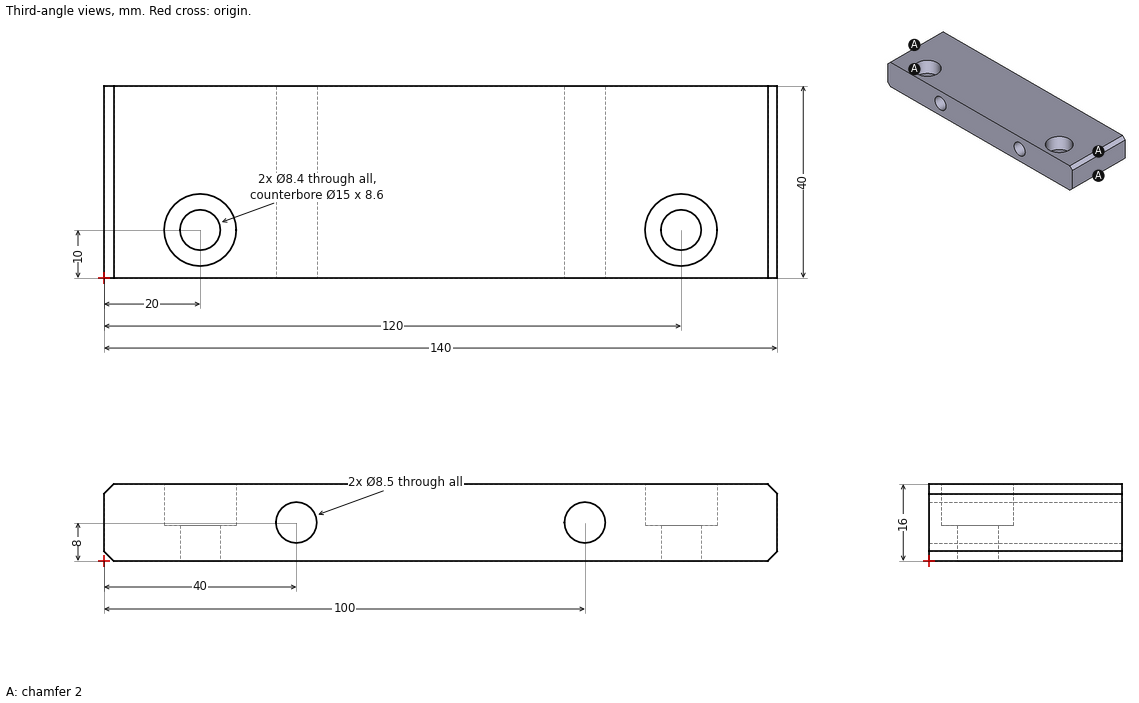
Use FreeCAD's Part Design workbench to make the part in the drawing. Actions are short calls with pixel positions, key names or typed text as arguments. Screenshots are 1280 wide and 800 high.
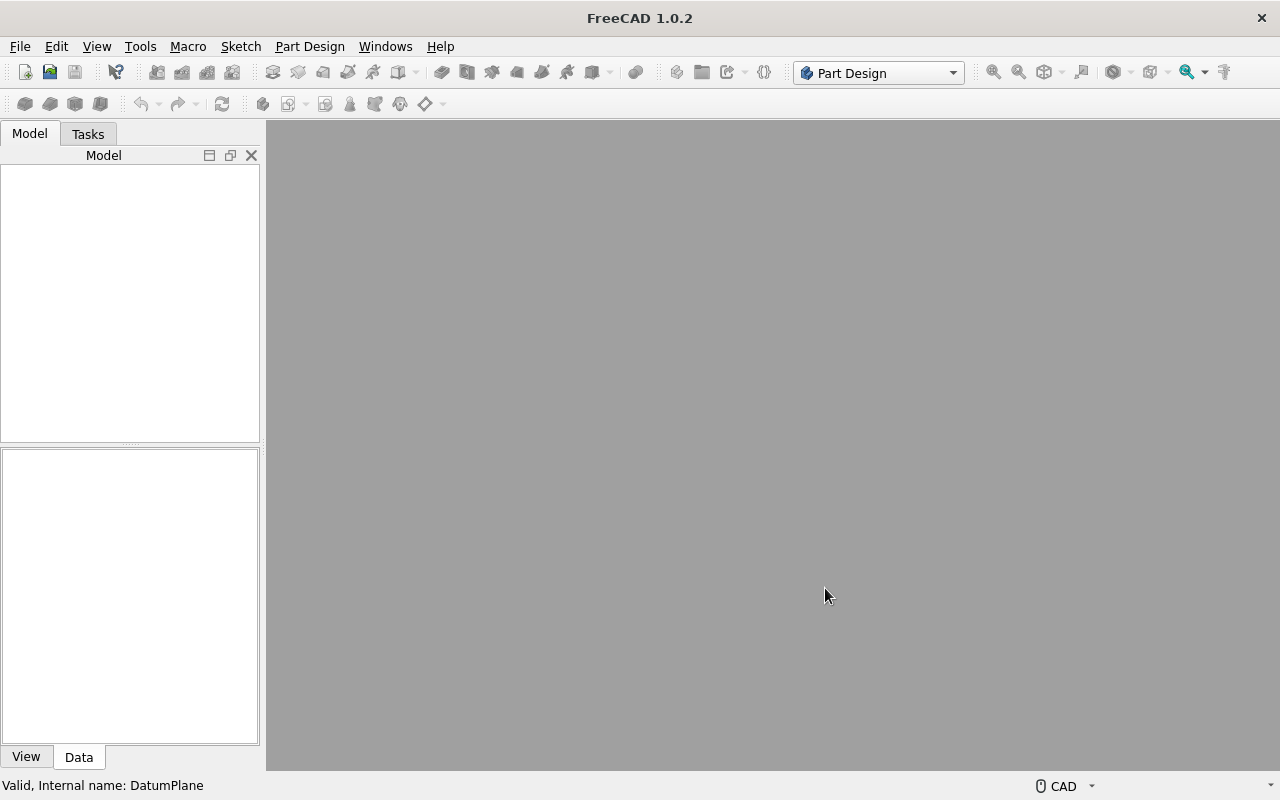
click(25, 72)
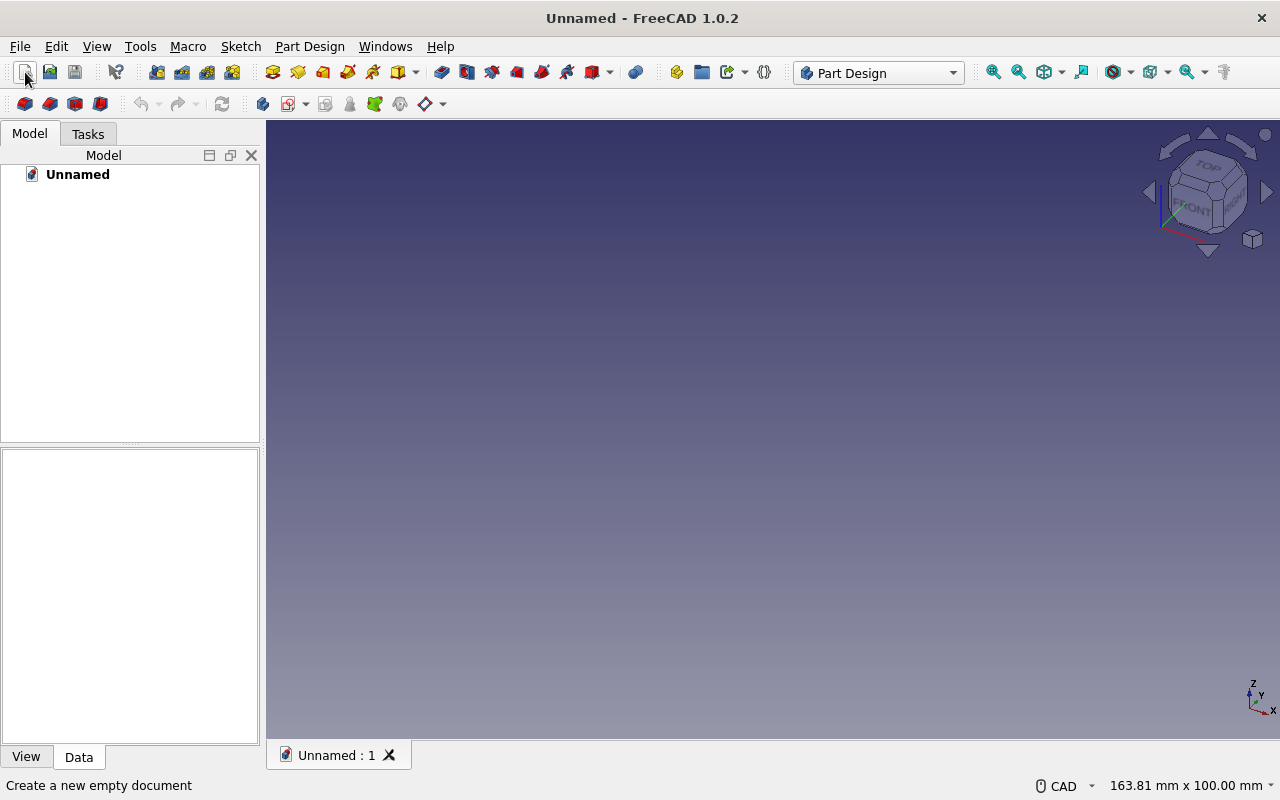
click(288, 104)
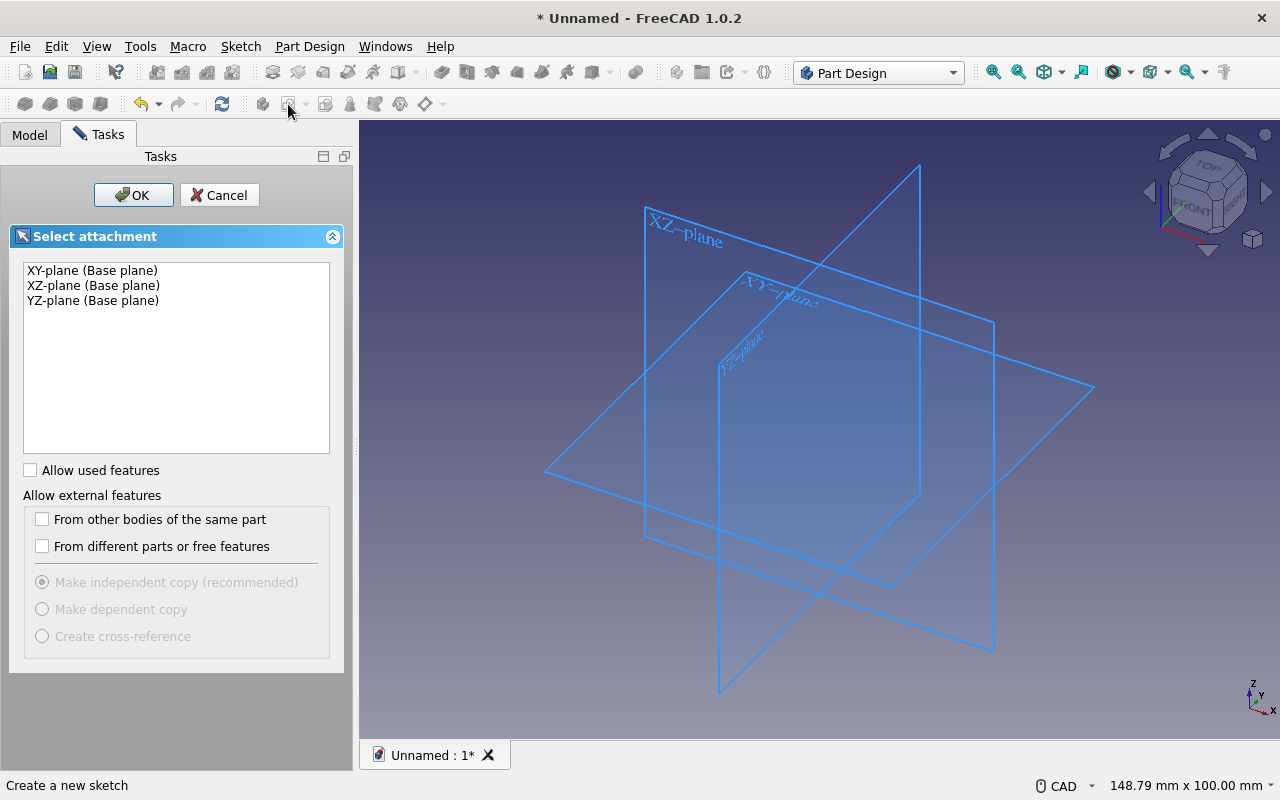
click(84, 270)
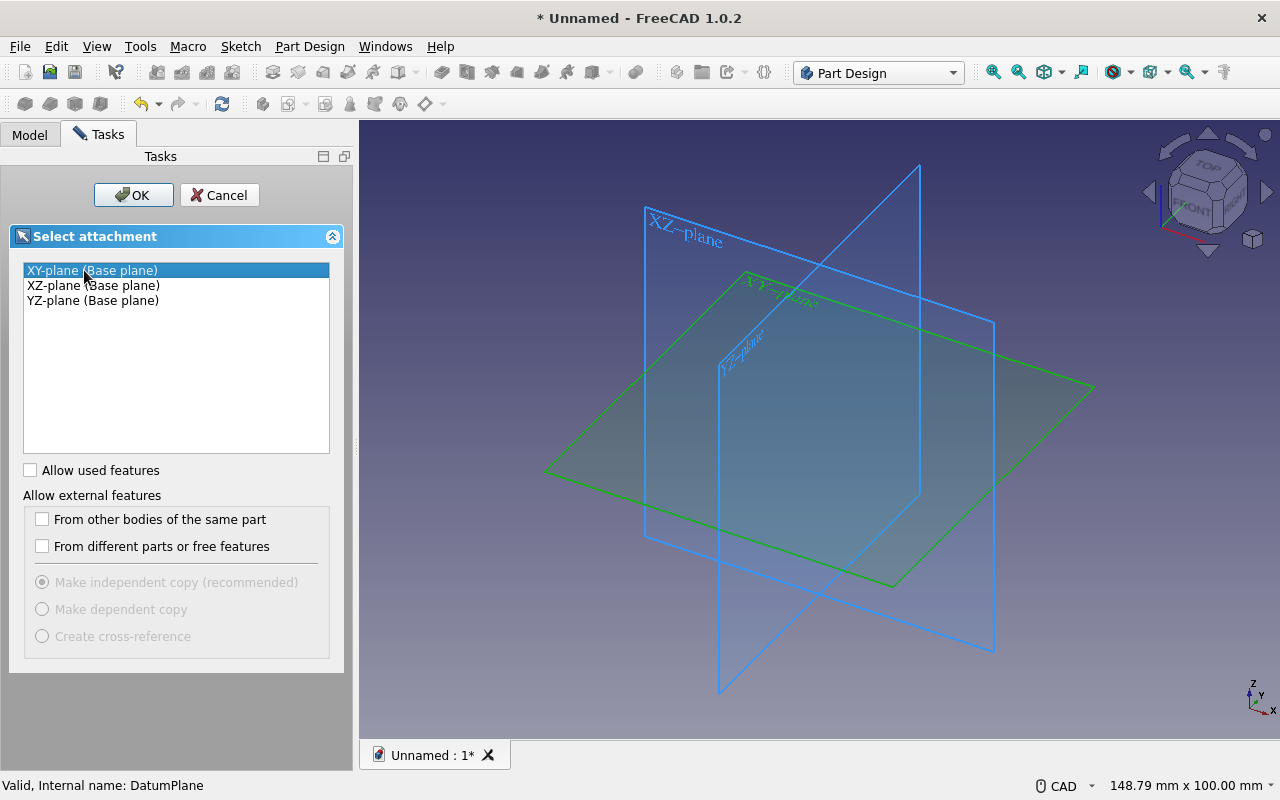
click(134, 195)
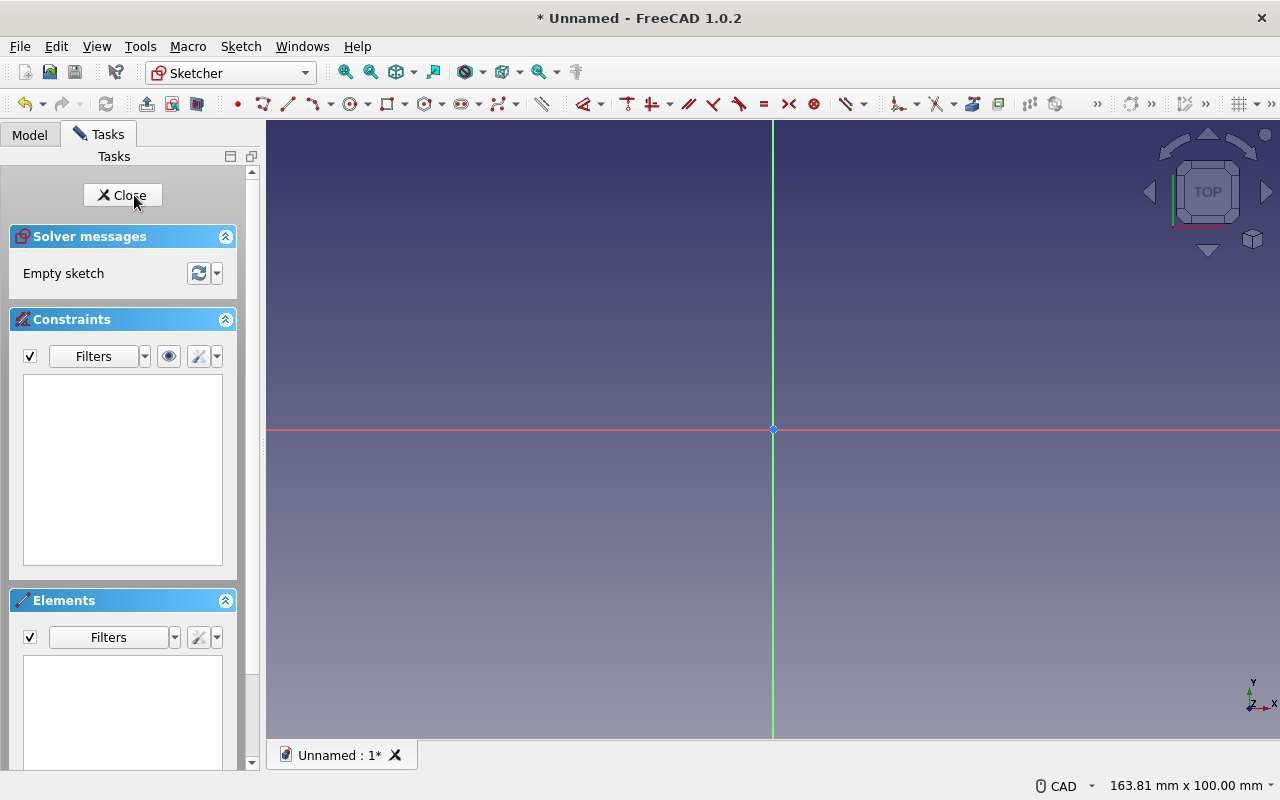
scroll(294, 580, down, 3)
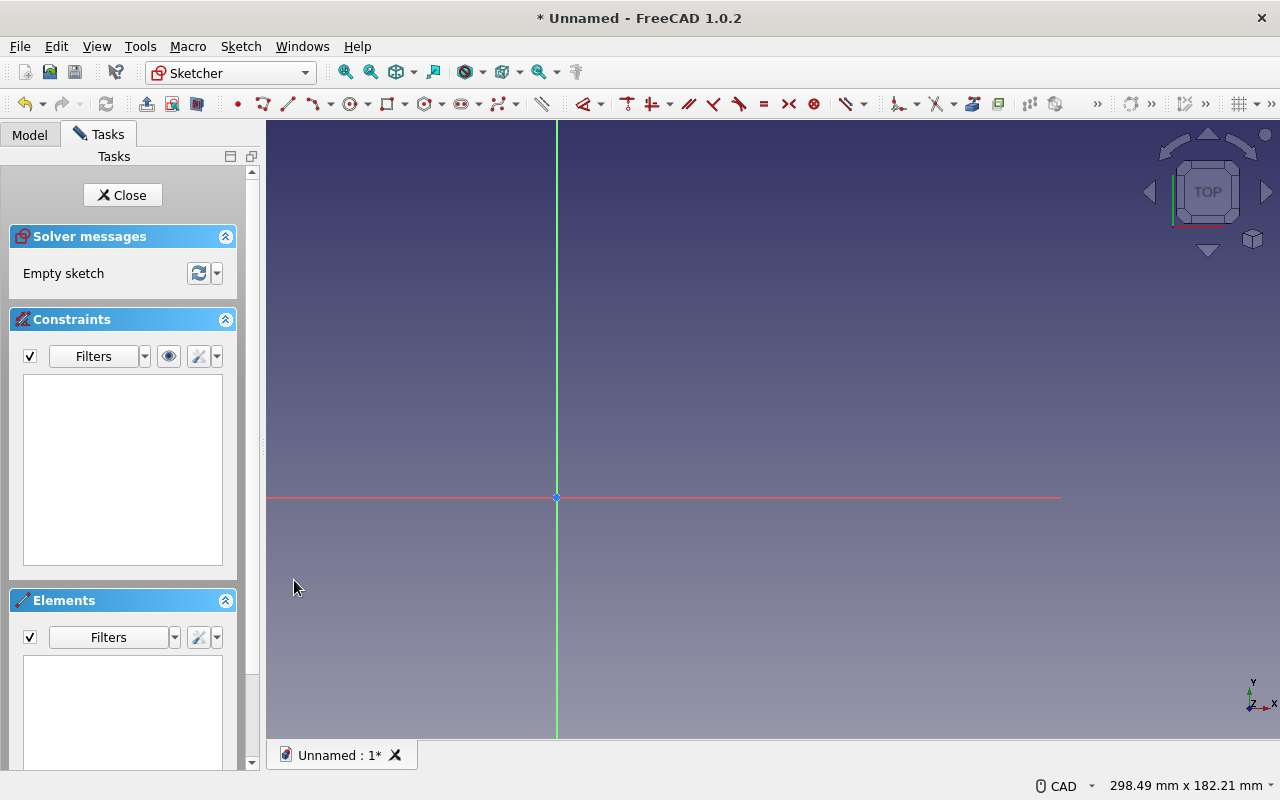
click(386, 104)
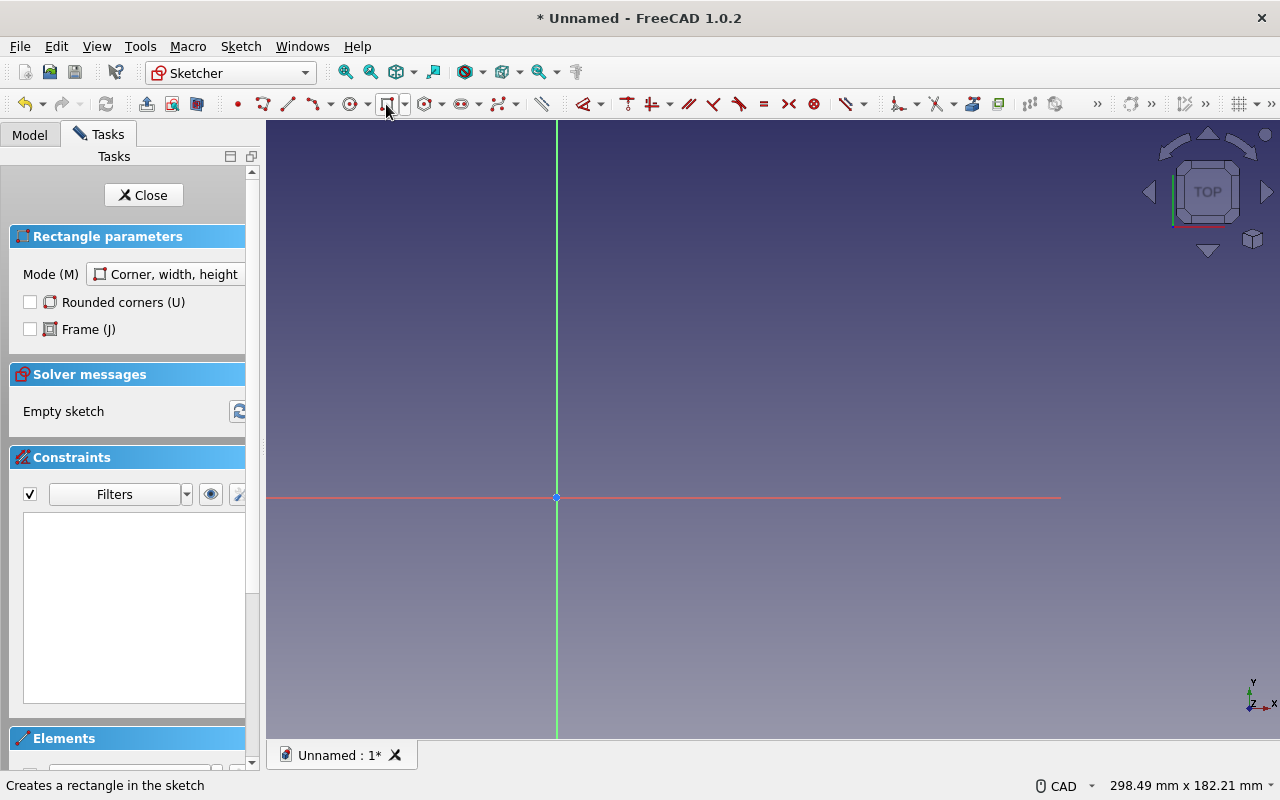
click(557, 498)
click(1032, 362)
key(Escape)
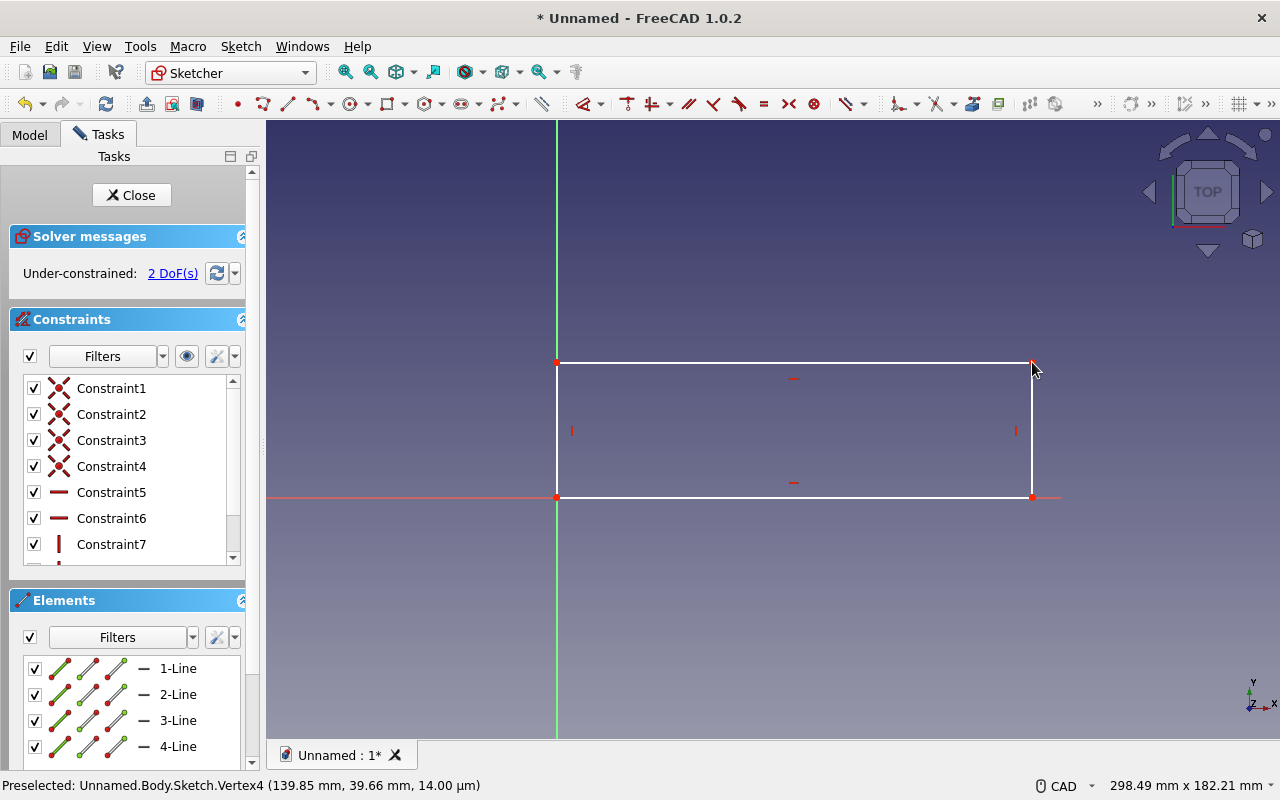
click(1032, 457)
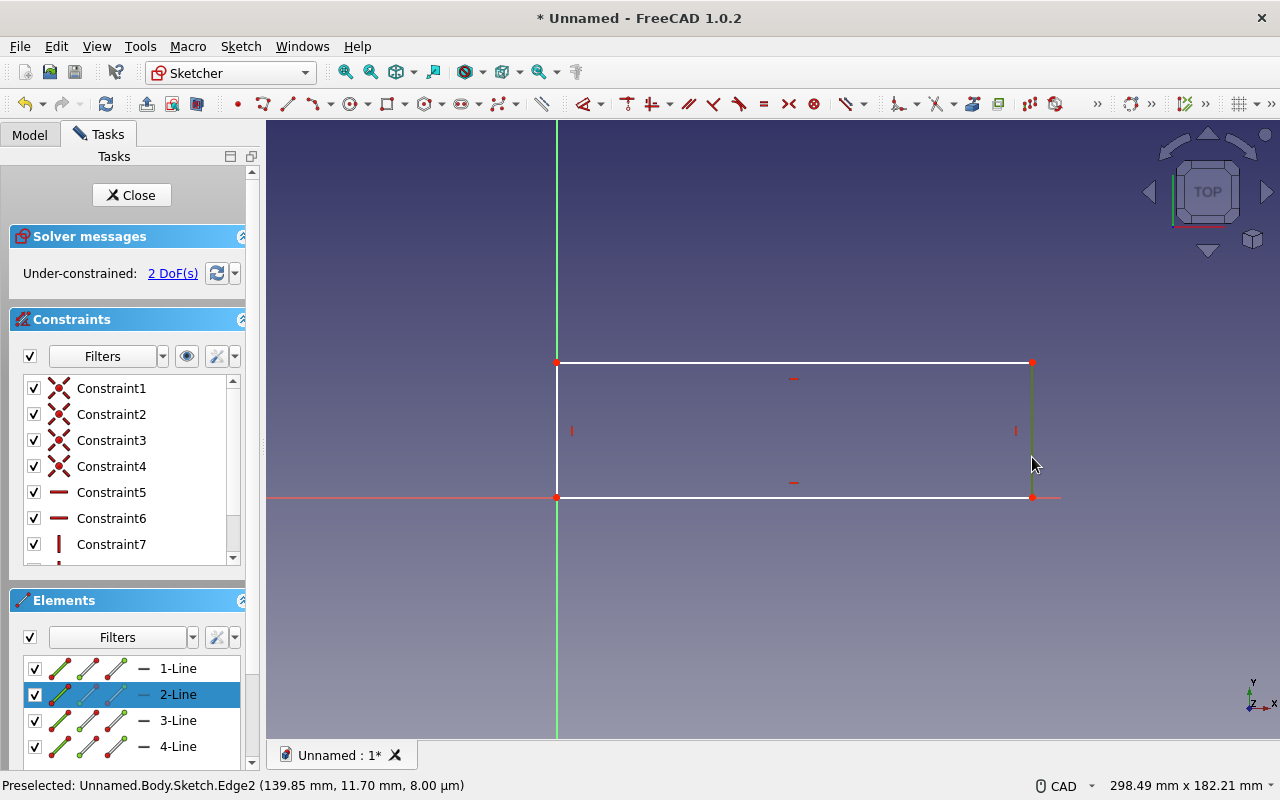
key(i)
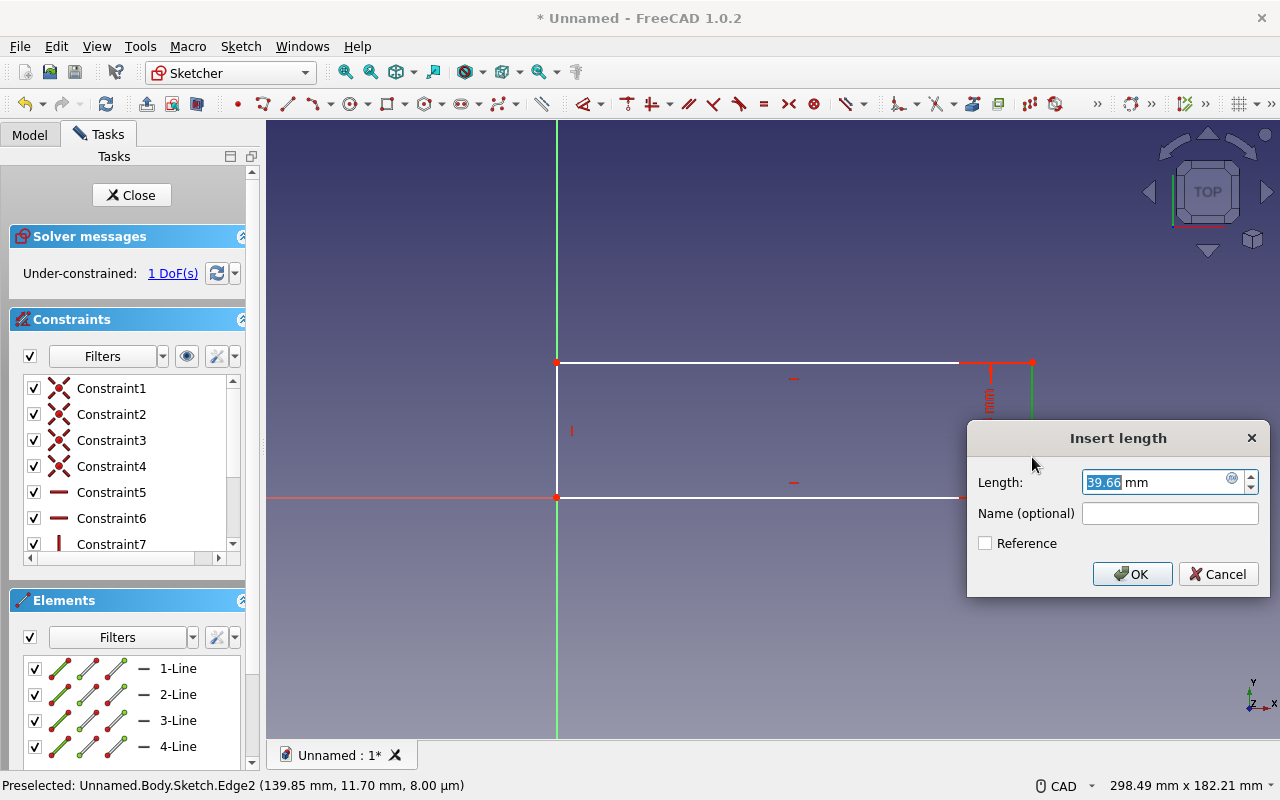
text(40)
key(Return)